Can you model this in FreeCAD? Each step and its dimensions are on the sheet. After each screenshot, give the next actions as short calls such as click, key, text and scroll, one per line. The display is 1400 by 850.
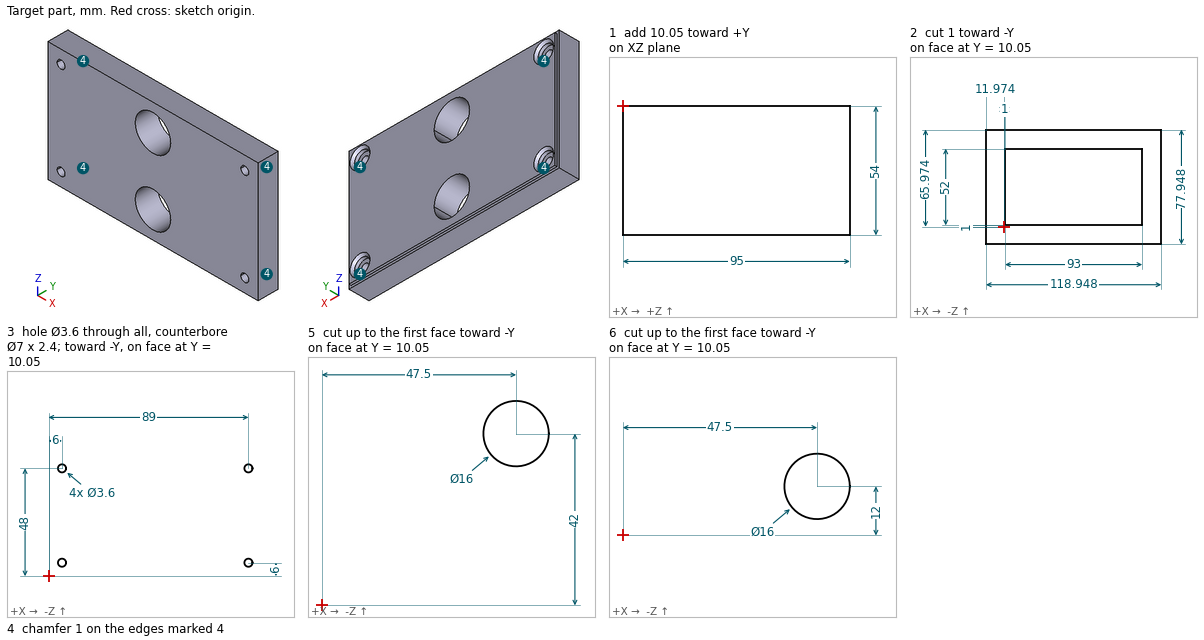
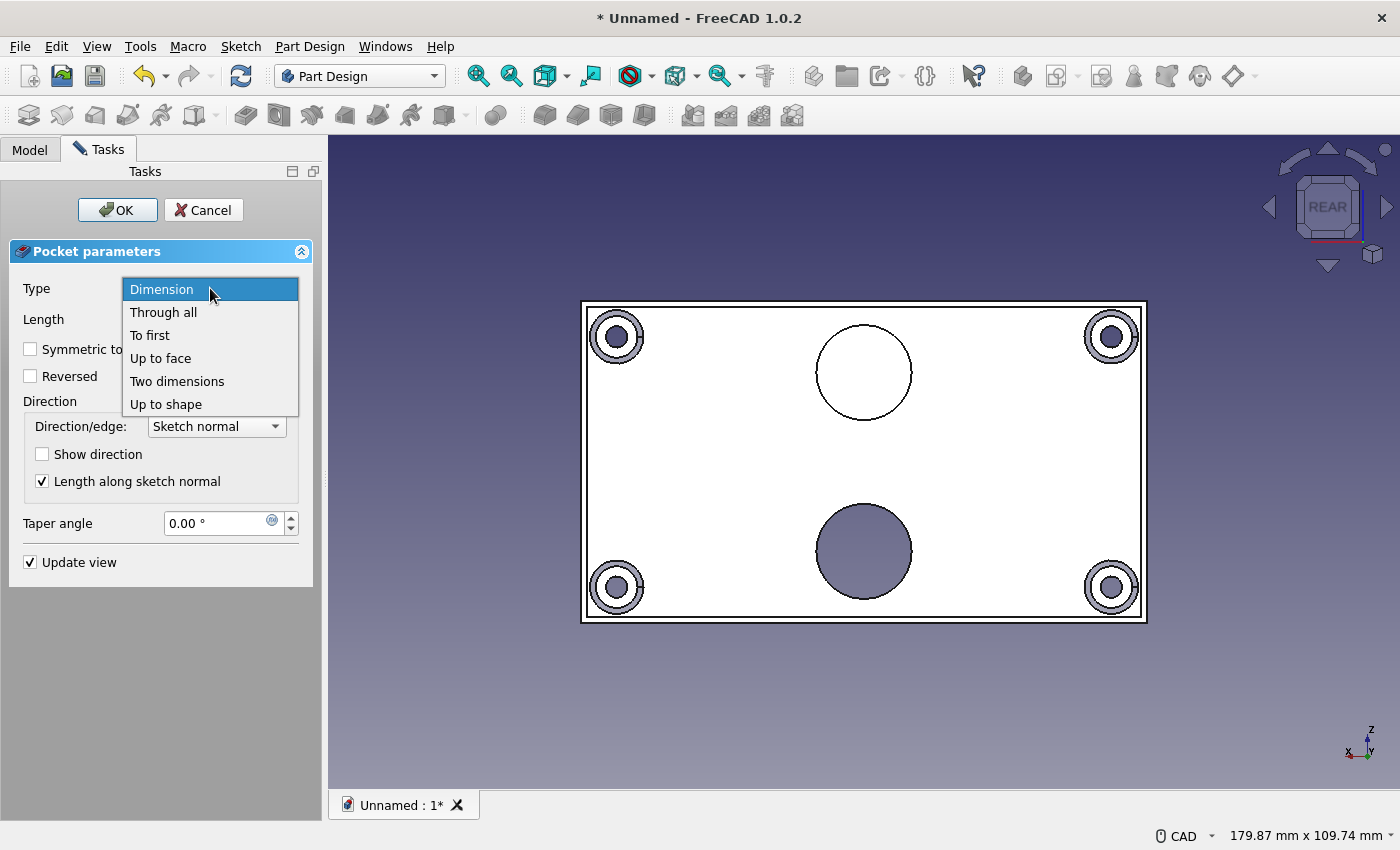
click(208, 336)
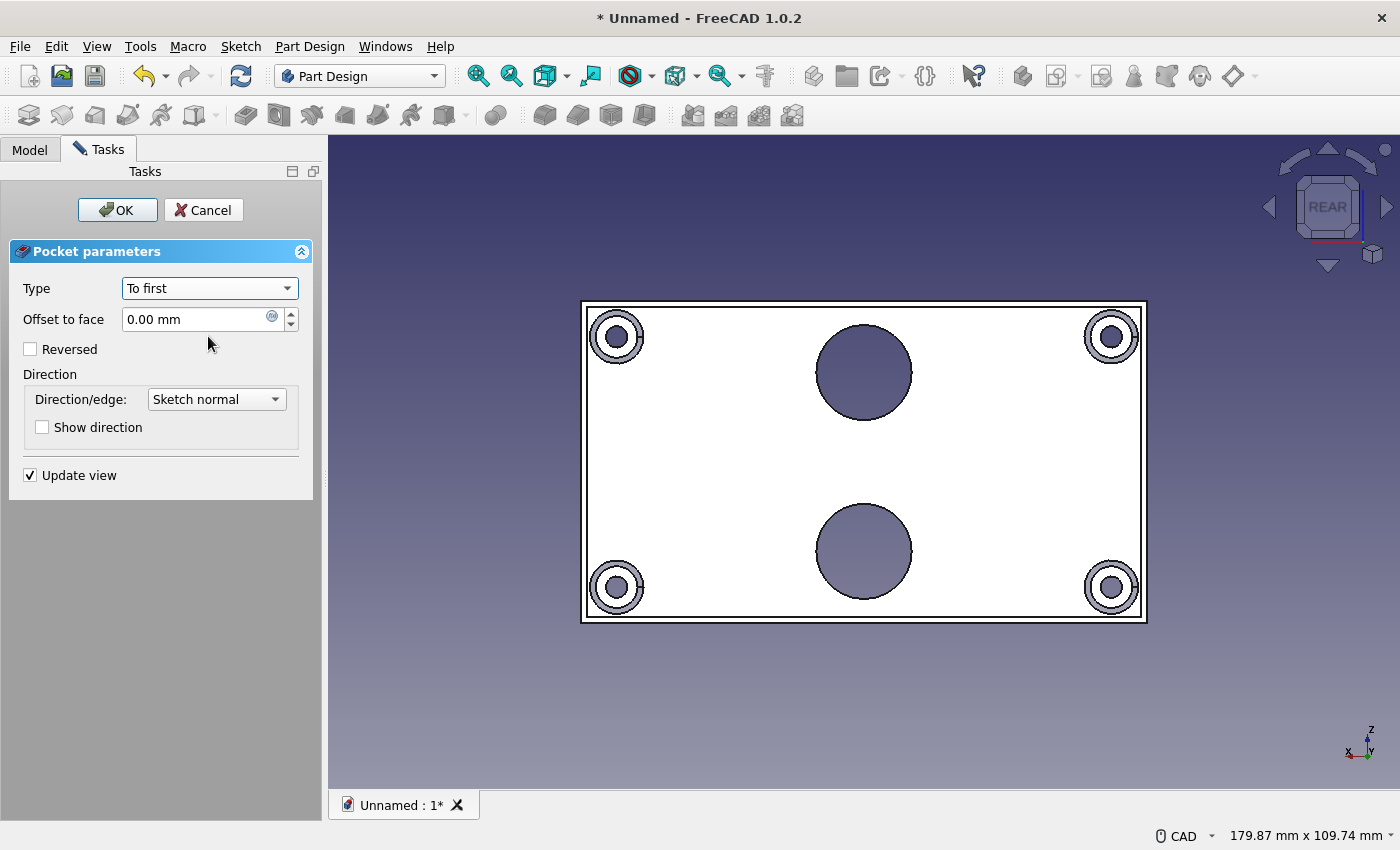
click(118, 210)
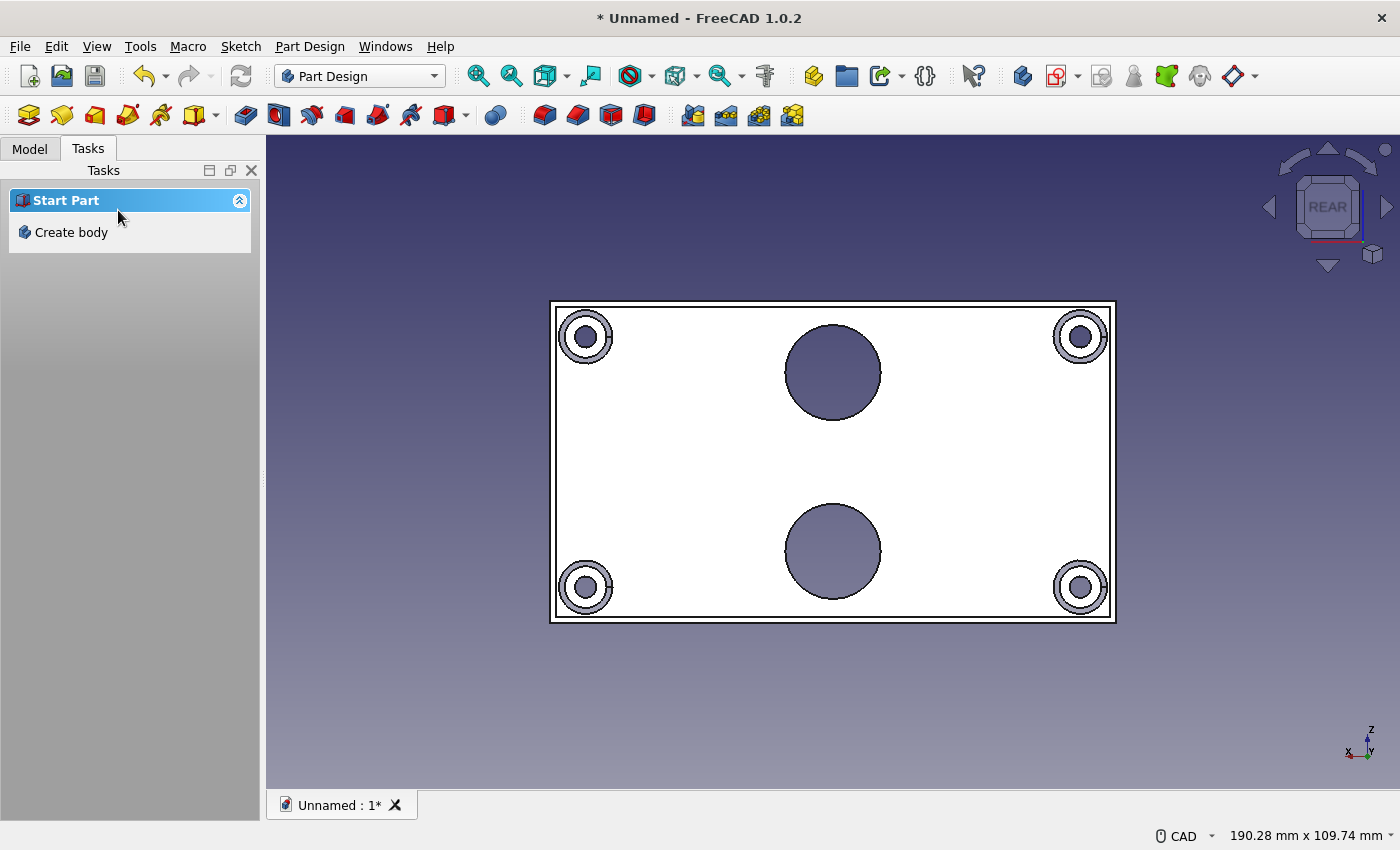
key(0)